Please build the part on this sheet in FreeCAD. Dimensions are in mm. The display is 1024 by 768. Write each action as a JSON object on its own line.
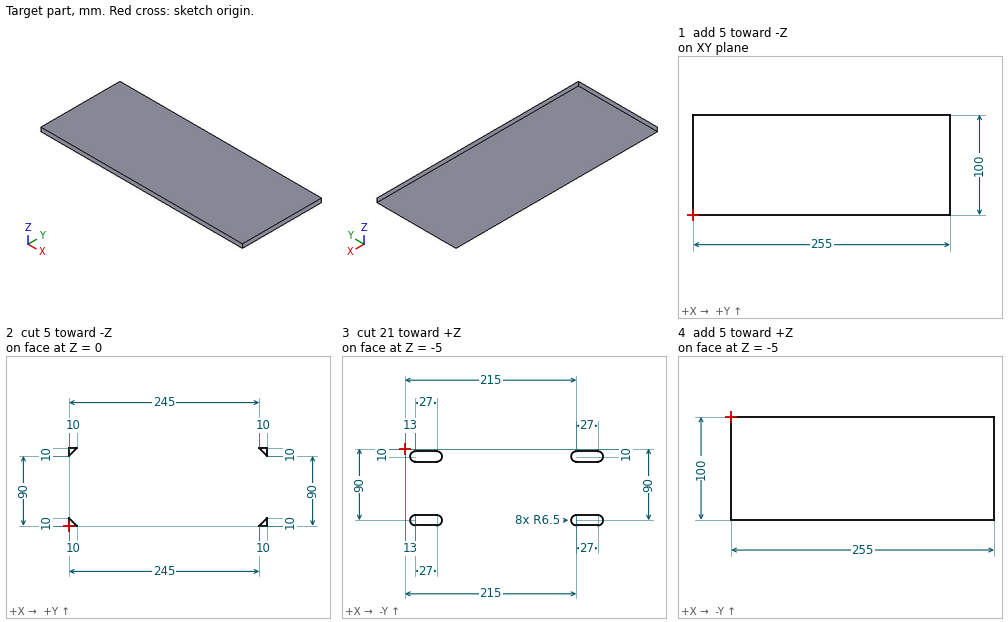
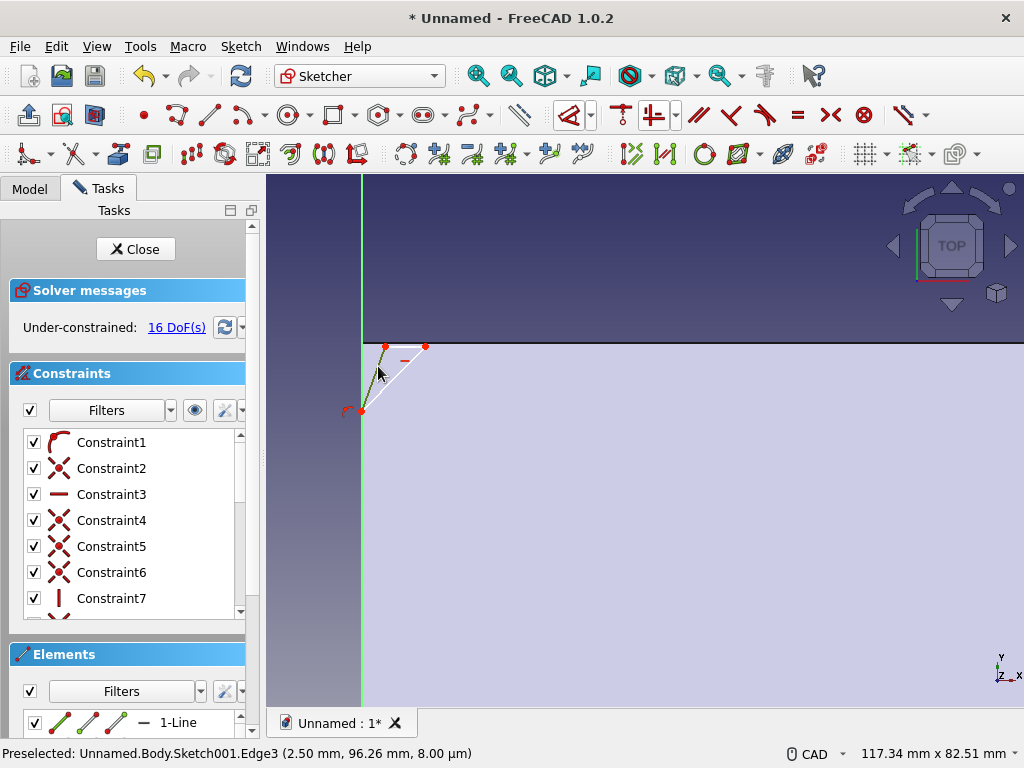
{"action": "key", "text": "v"}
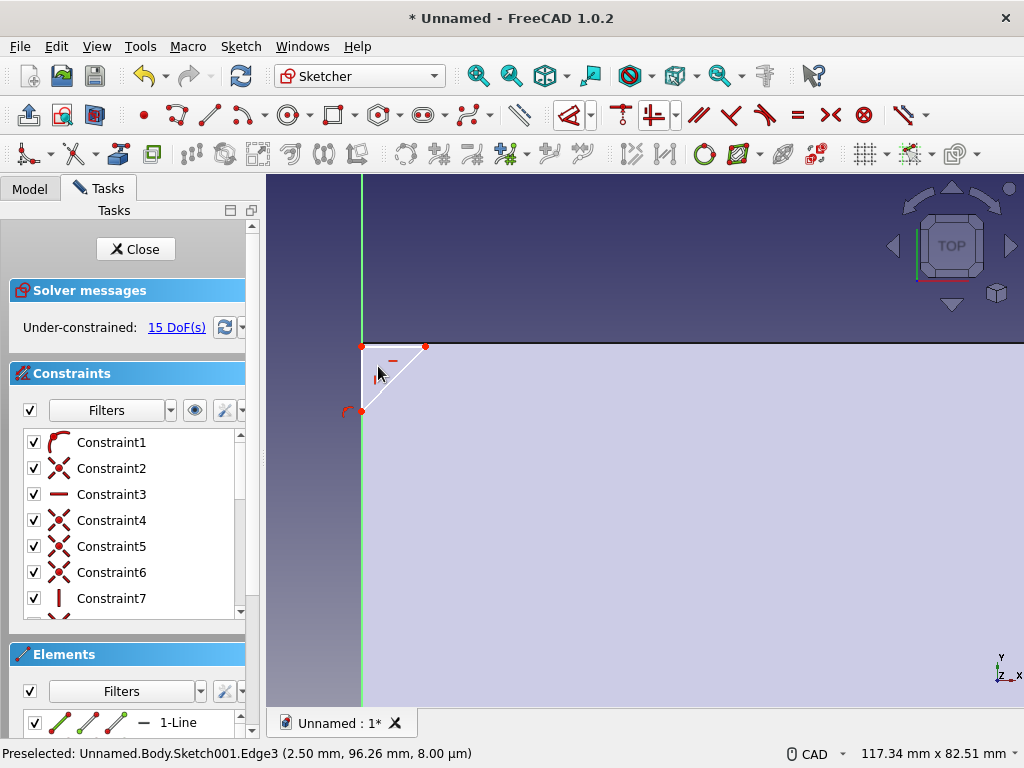
{"action": "scroll", "coordinate": [377, 367], "scroll_direction": "down", "scroll_amount": 7}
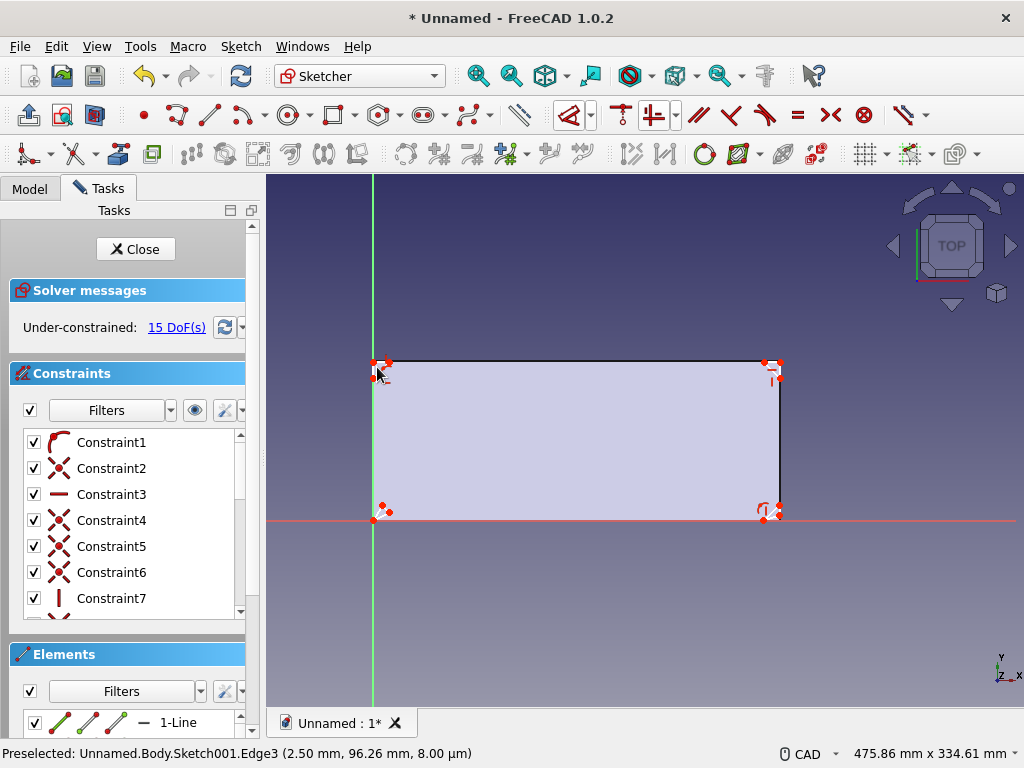
{"action": "scroll", "coordinate": [775, 517], "scroll_direction": "up", "scroll_amount": 7}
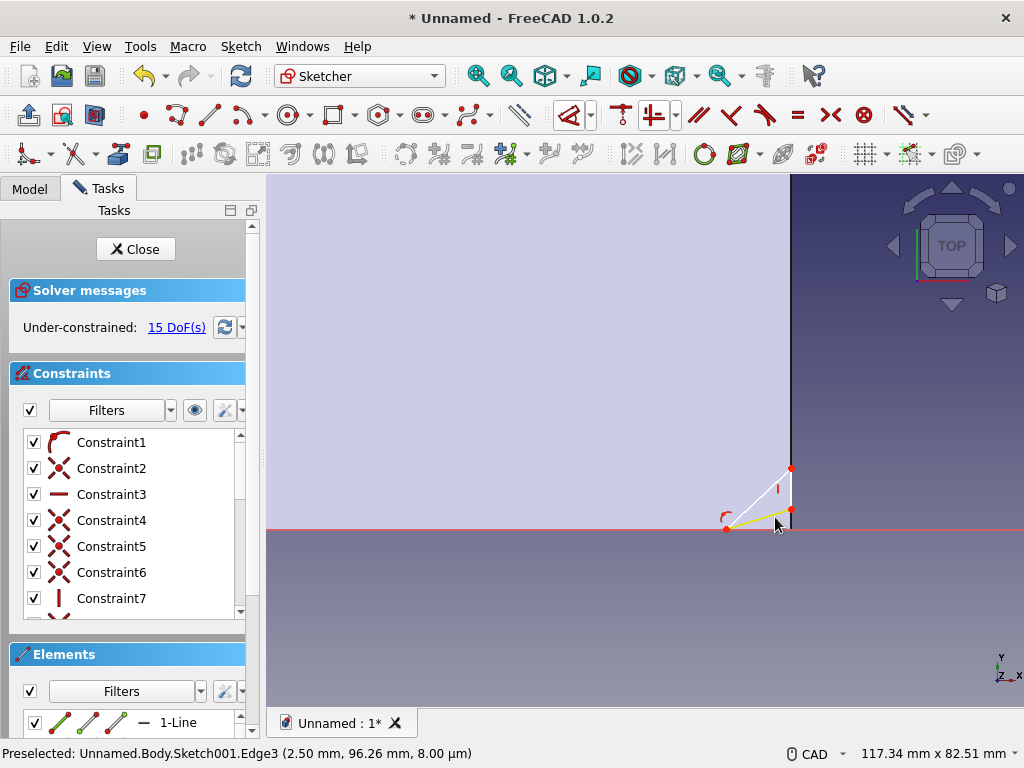
{"action": "left_click", "coordinate": [772, 515]}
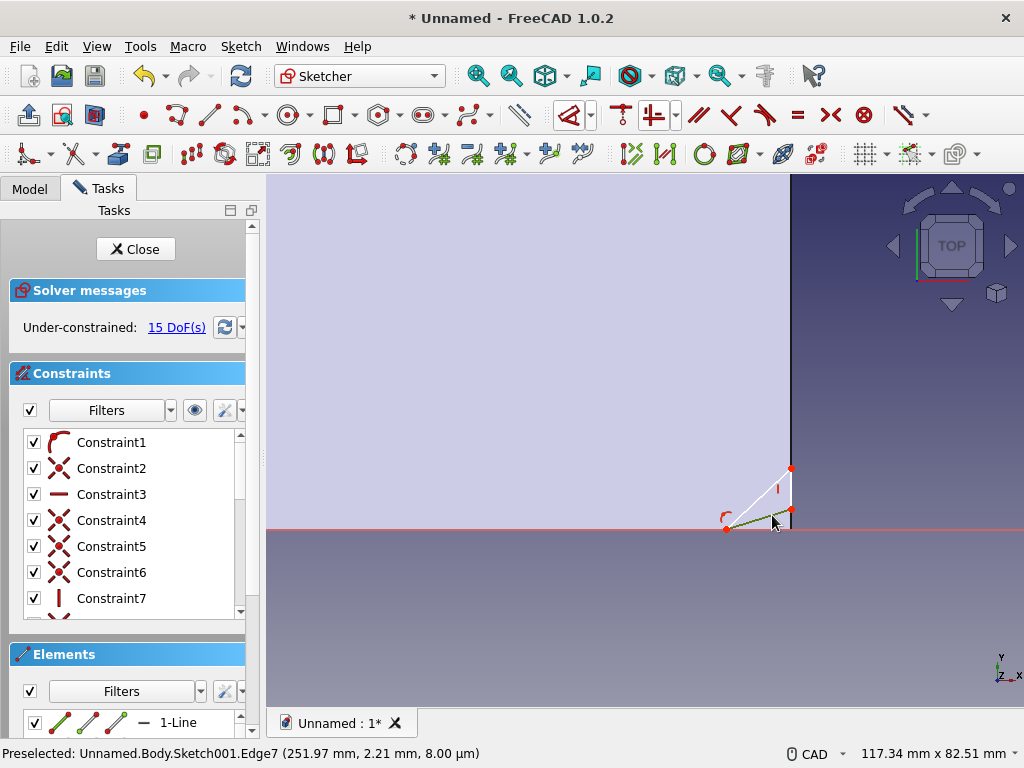
{"action": "key", "text": "h"}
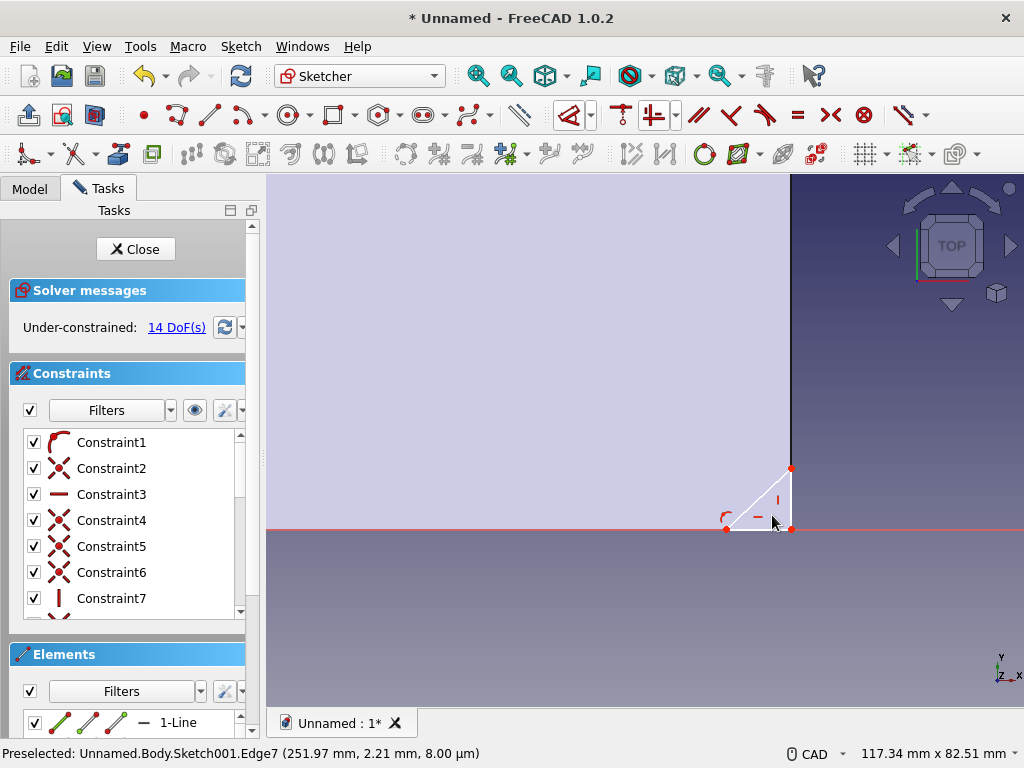
{"action": "scroll", "coordinate": [776, 517], "scroll_direction": "down", "scroll_amount": 7}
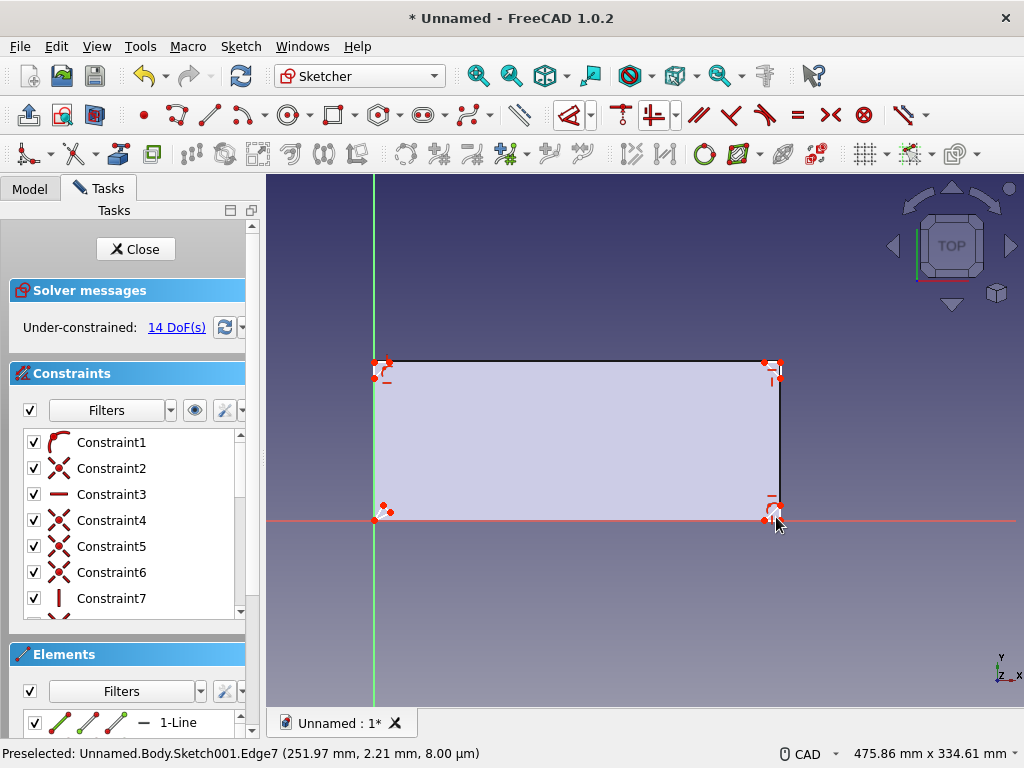
{"action": "scroll", "coordinate": [379, 518], "scroll_direction": "up", "scroll_amount": 10}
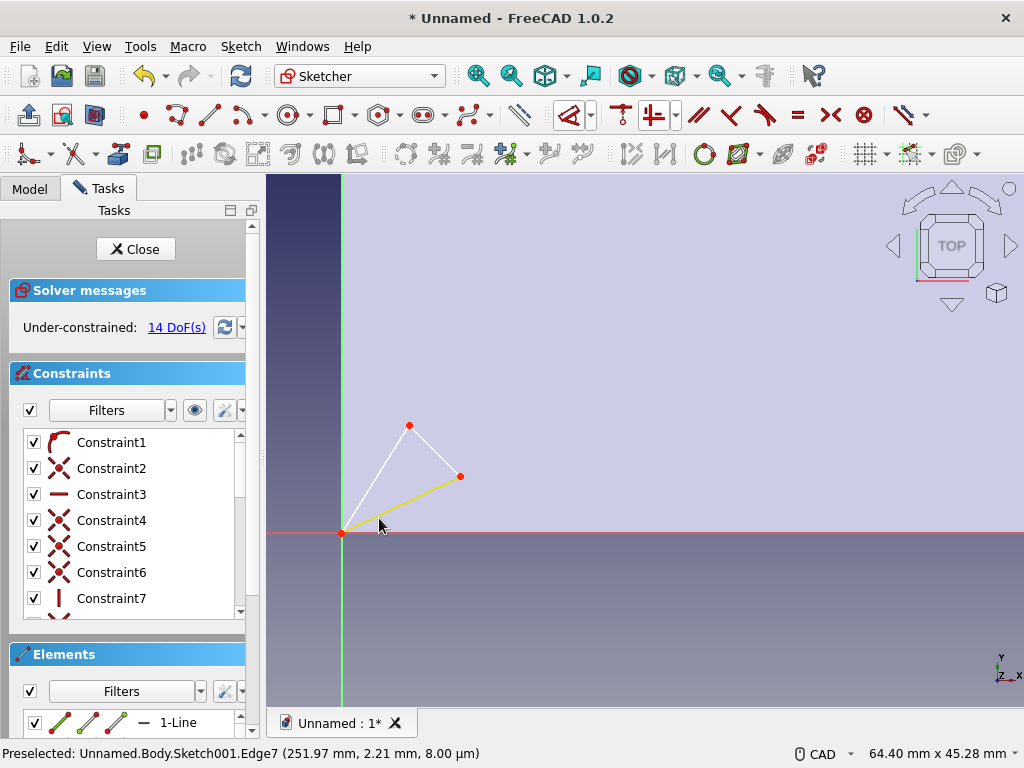
{"action": "left_click", "coordinate": [378, 516]}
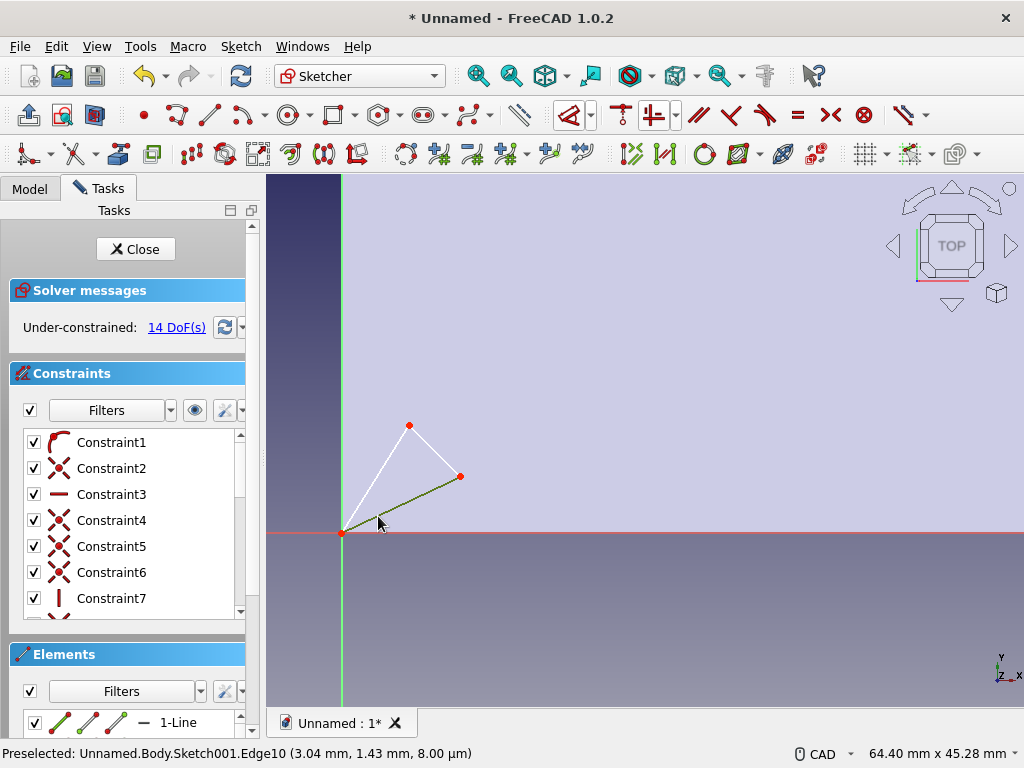
{"action": "key", "text": "h"}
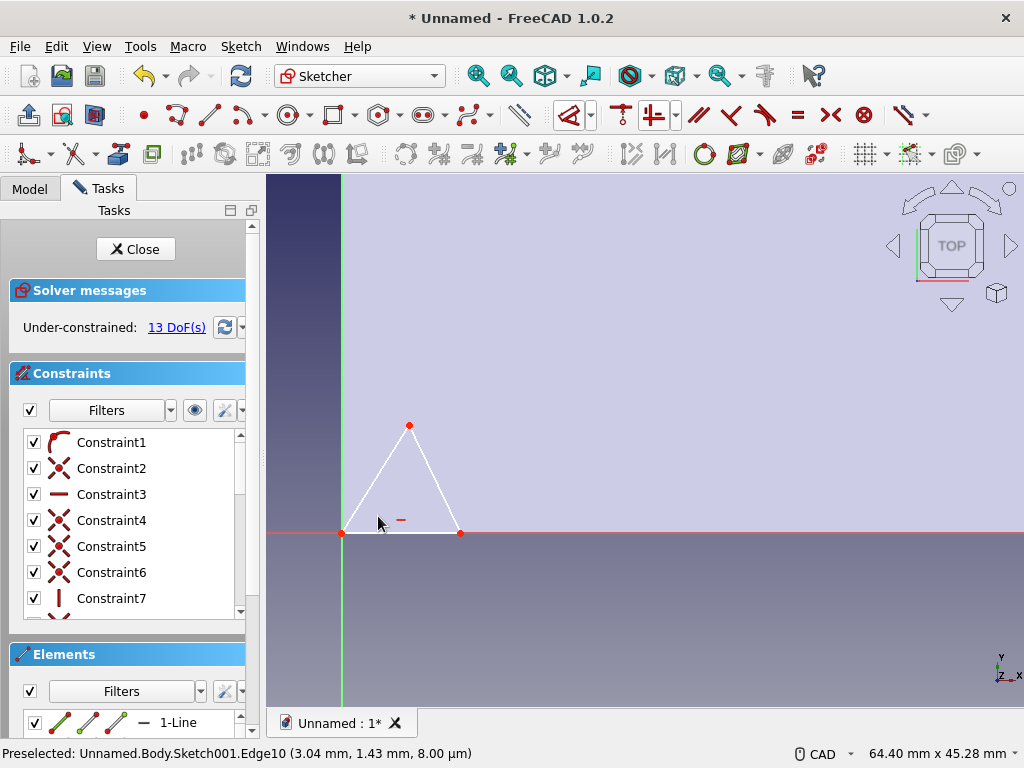
{"action": "left_click", "coordinate": [389, 458]}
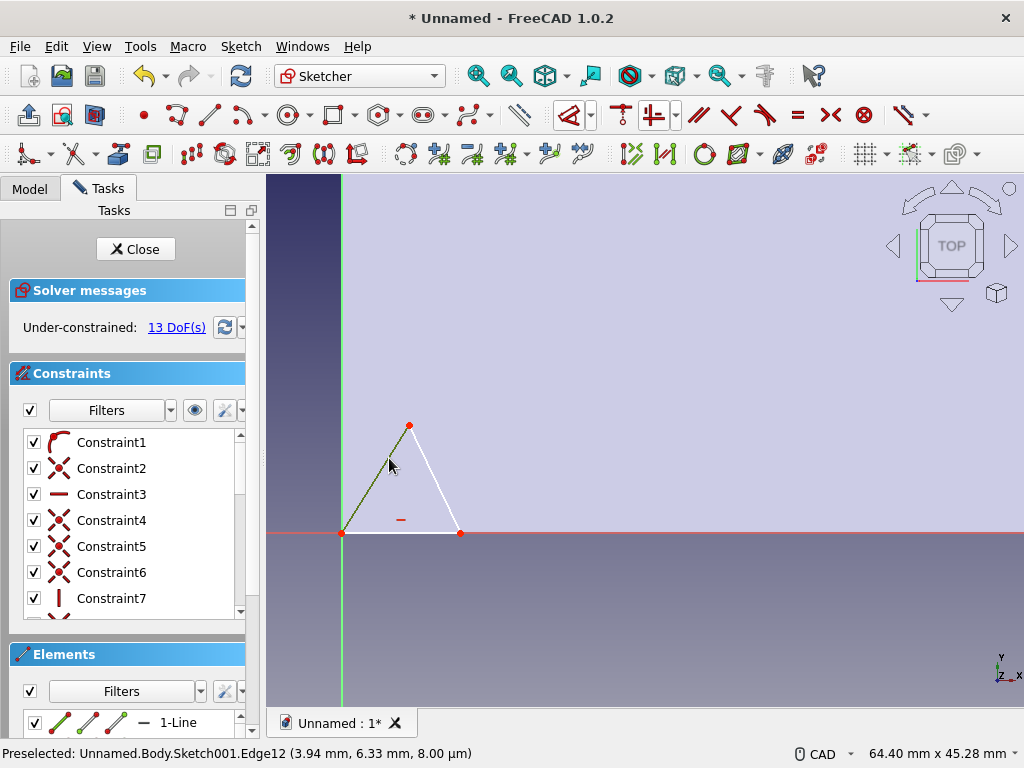
{"action": "key", "text": "v"}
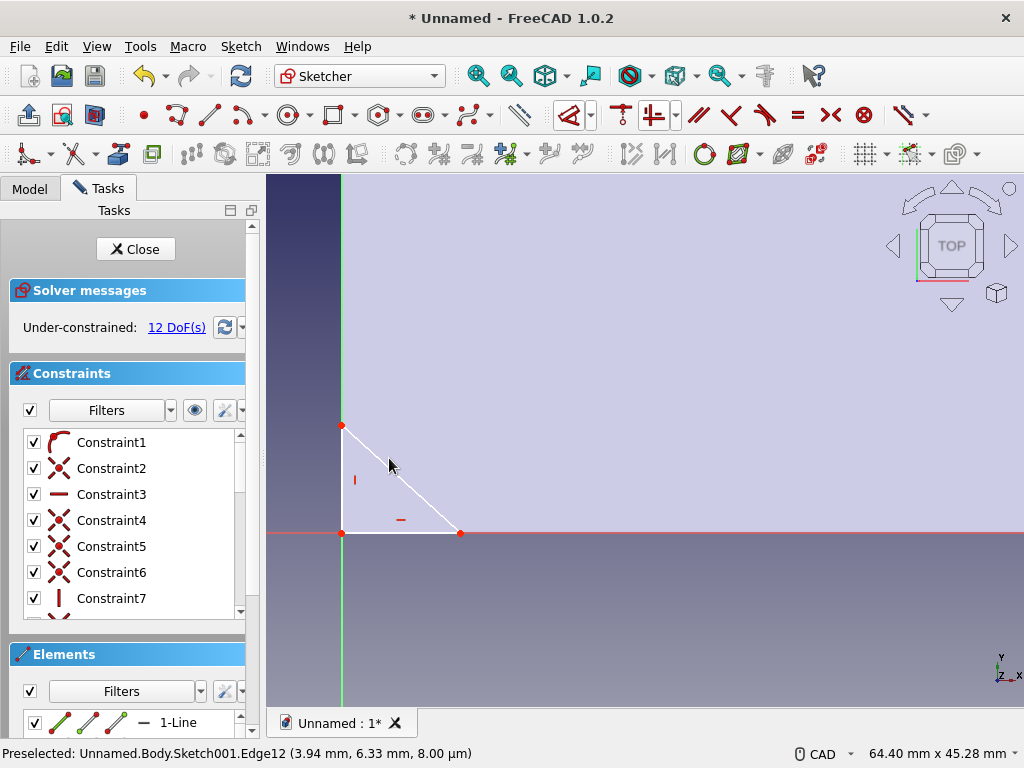
{"action": "key", "text": "d"}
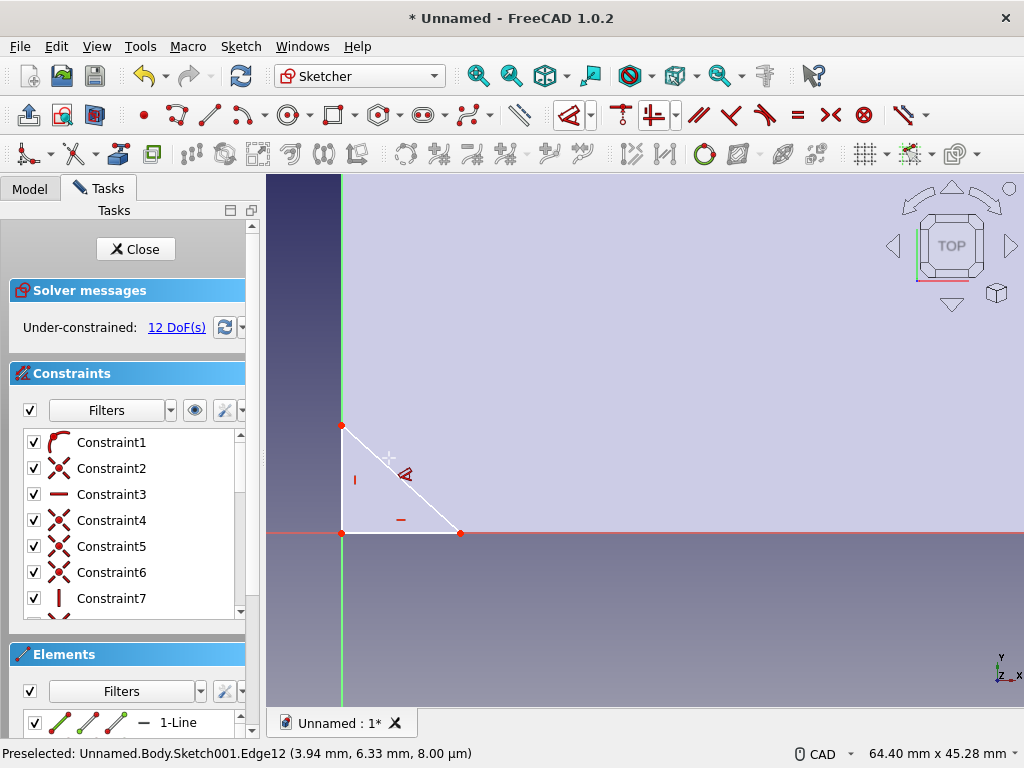
{"action": "scroll", "coordinate": [378, 518], "scroll_direction": "down", "scroll_amount": 10}